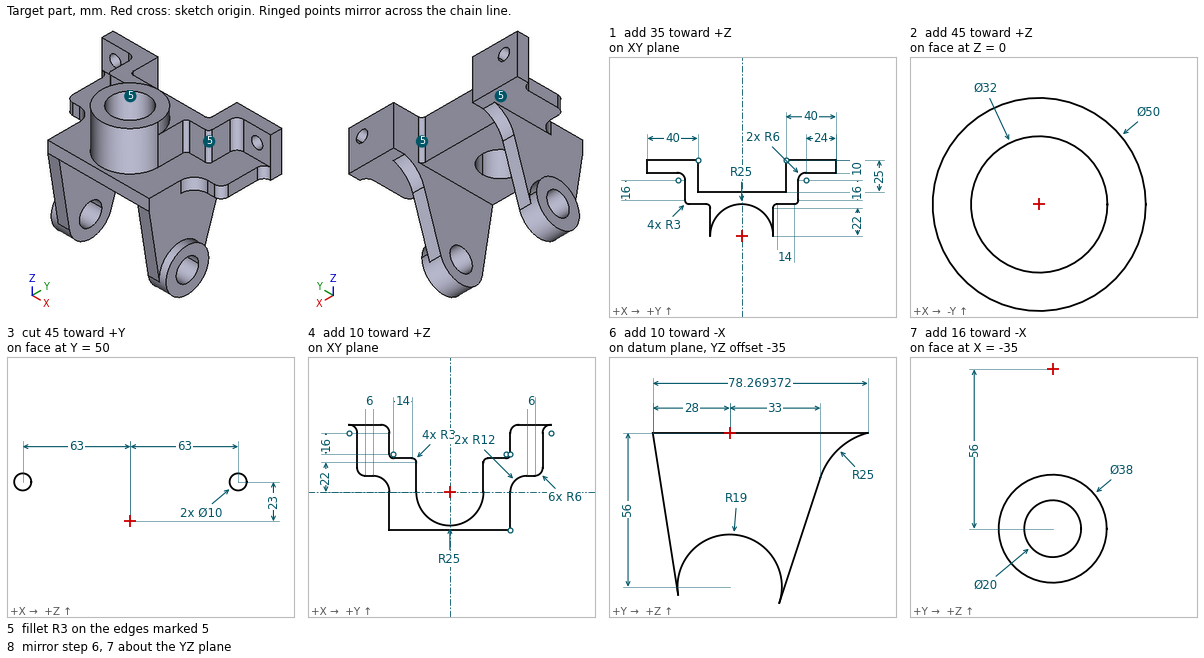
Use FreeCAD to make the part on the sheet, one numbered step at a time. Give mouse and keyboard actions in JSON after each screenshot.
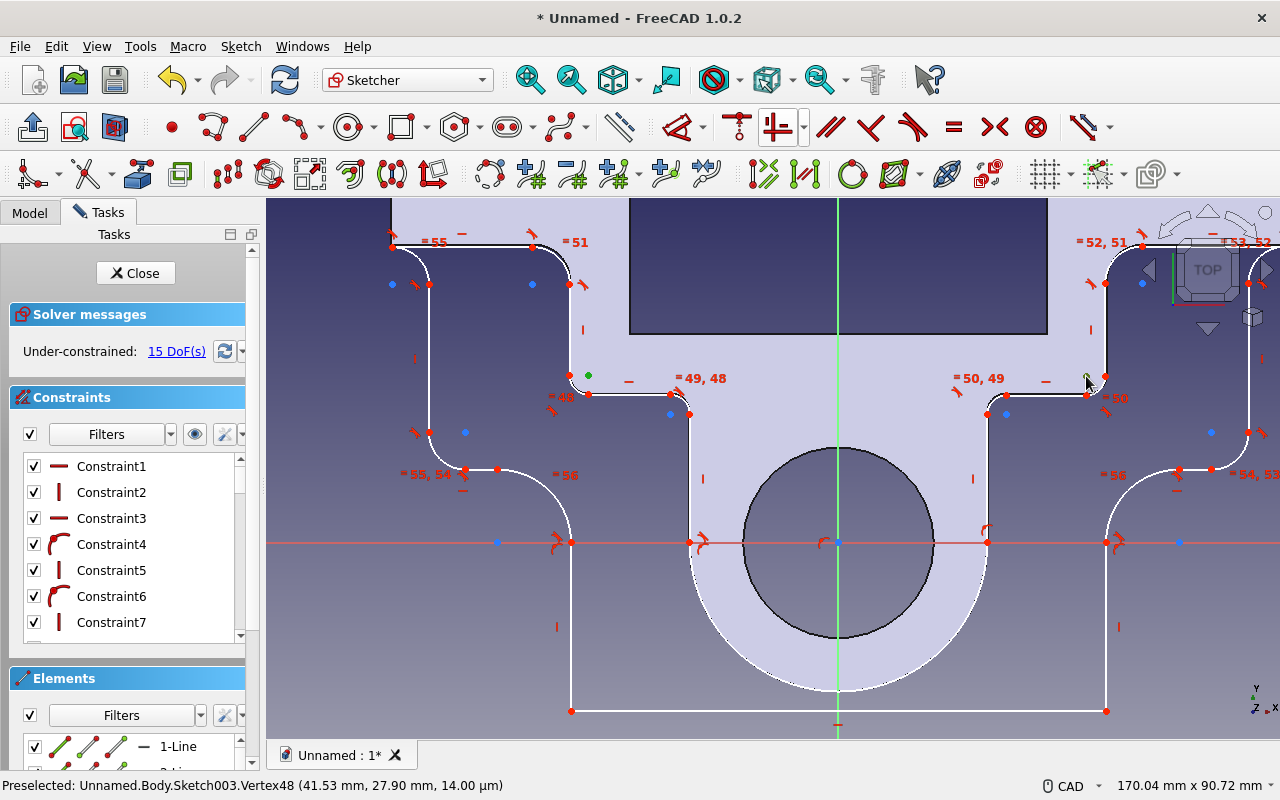
{"action": "left_click", "coordinate": [838, 642]}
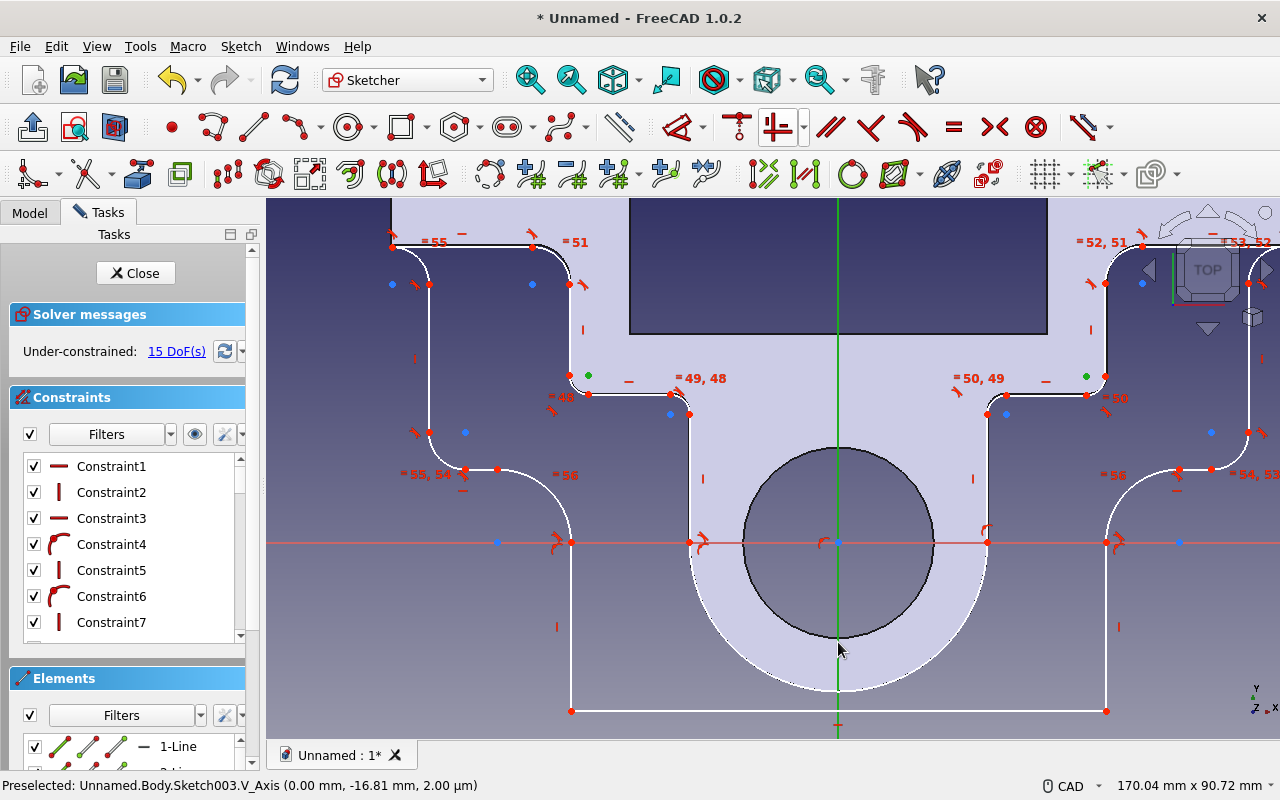
{"action": "left_click", "coordinate": [995, 128]}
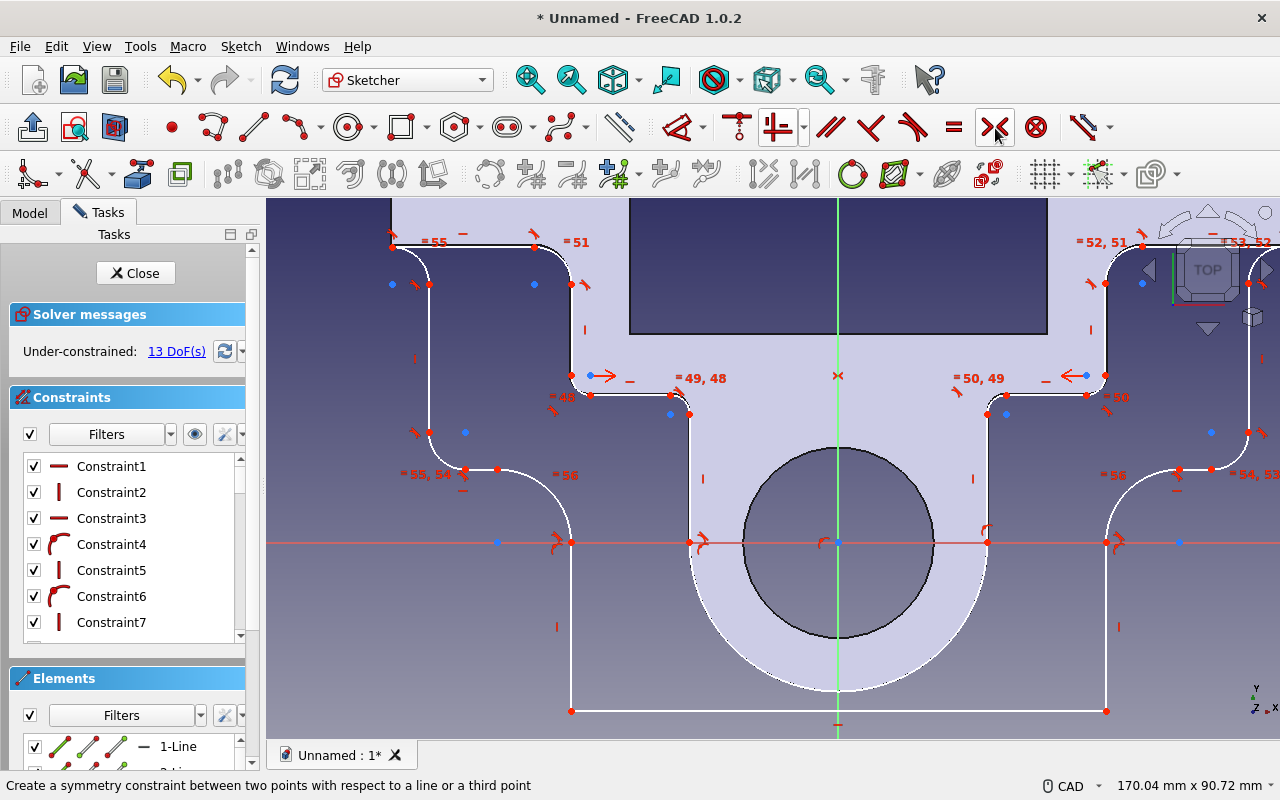
{"action": "scroll", "coordinate": [432, 451], "scroll_direction": "down", "scroll_amount": 2}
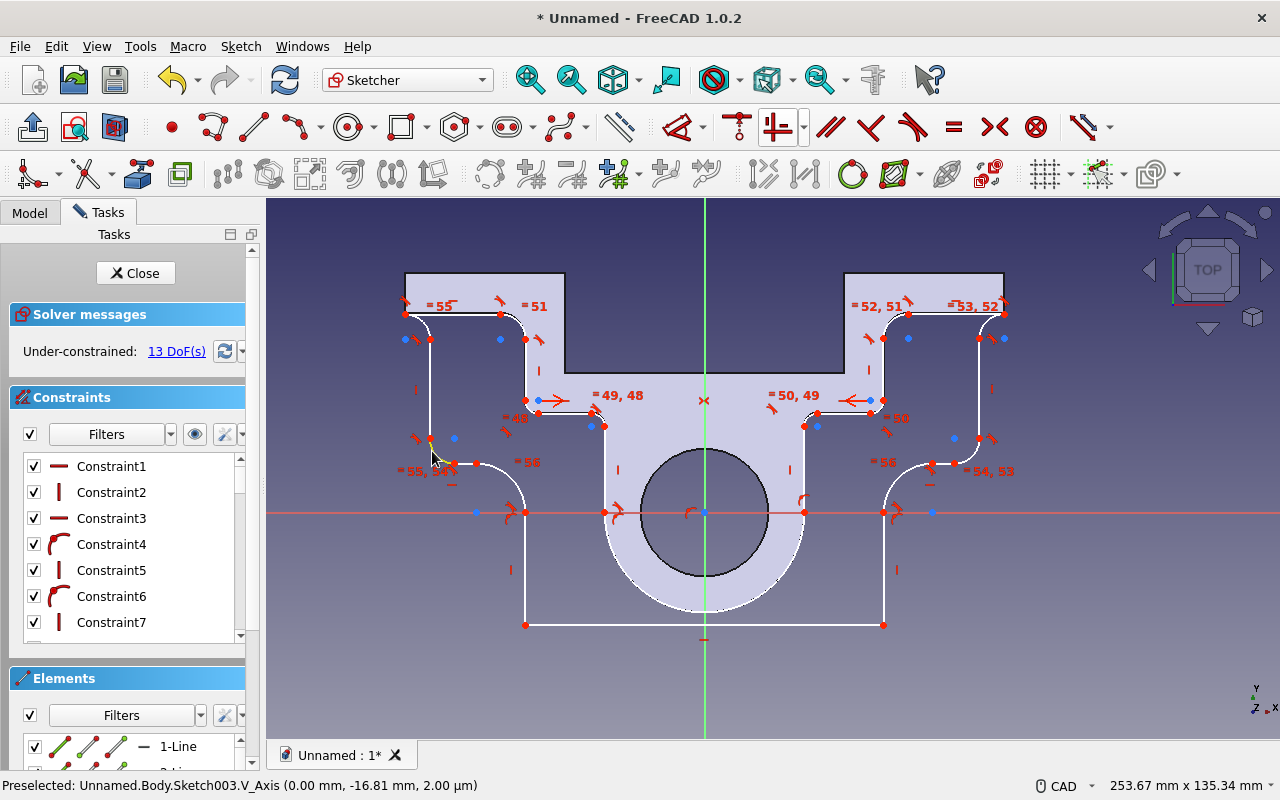
{"action": "left_click", "coordinate": [1004, 339]}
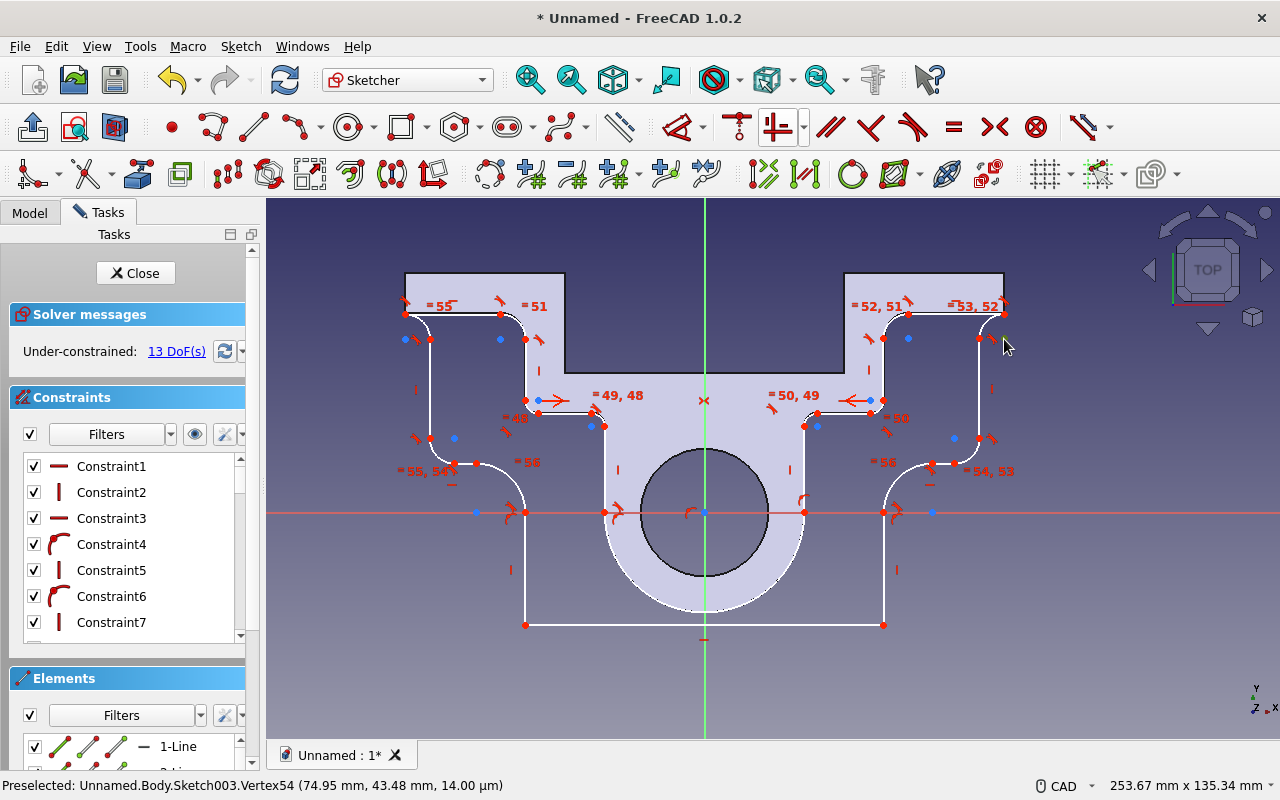
{"action": "left_click", "coordinate": [405, 339]}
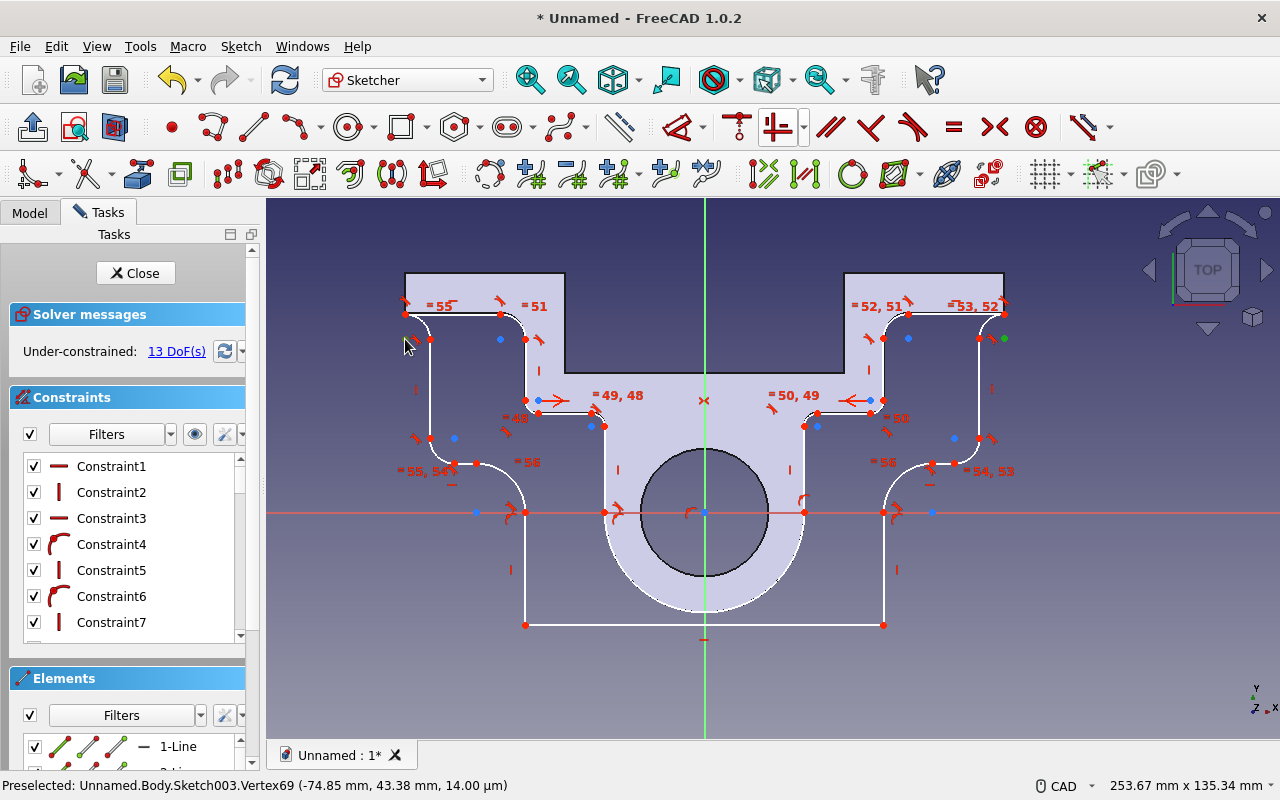
{"action": "left_click", "coordinate": [705, 676]}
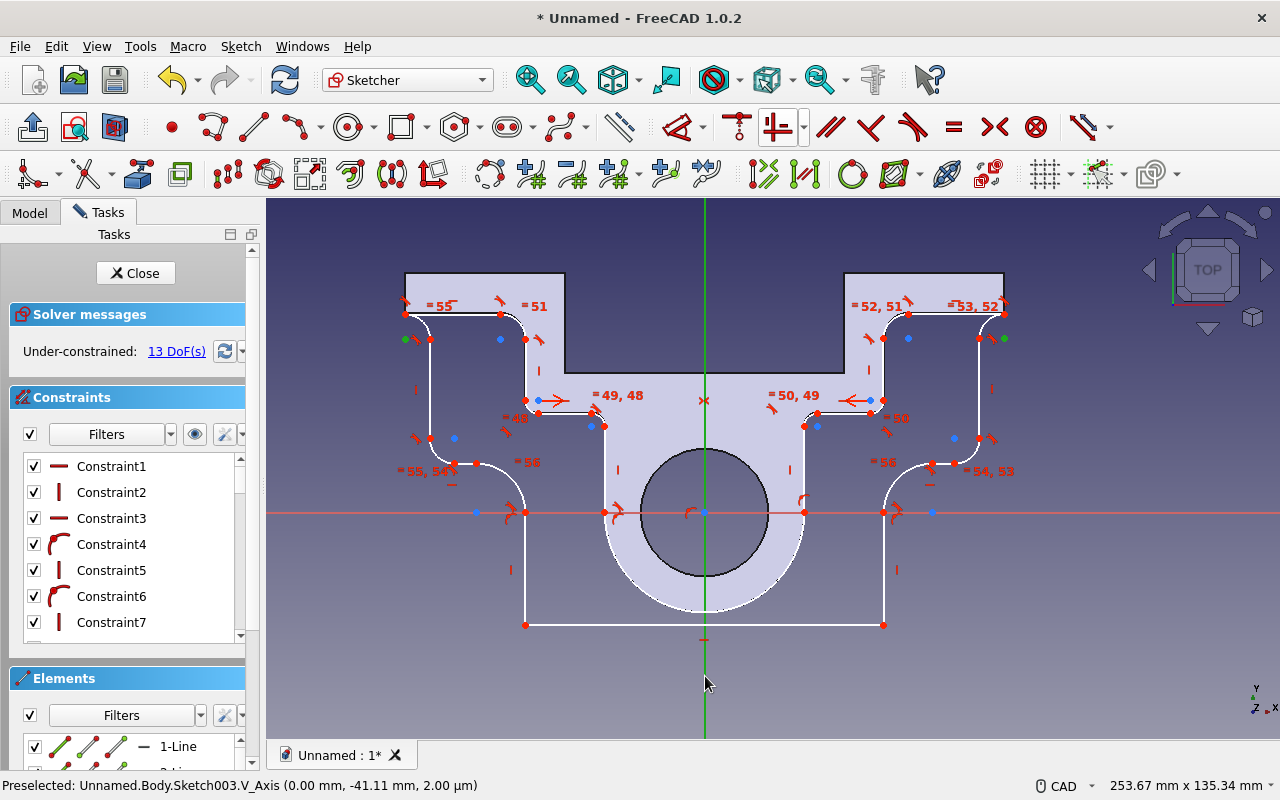
{"action": "left_click", "coordinate": [995, 128]}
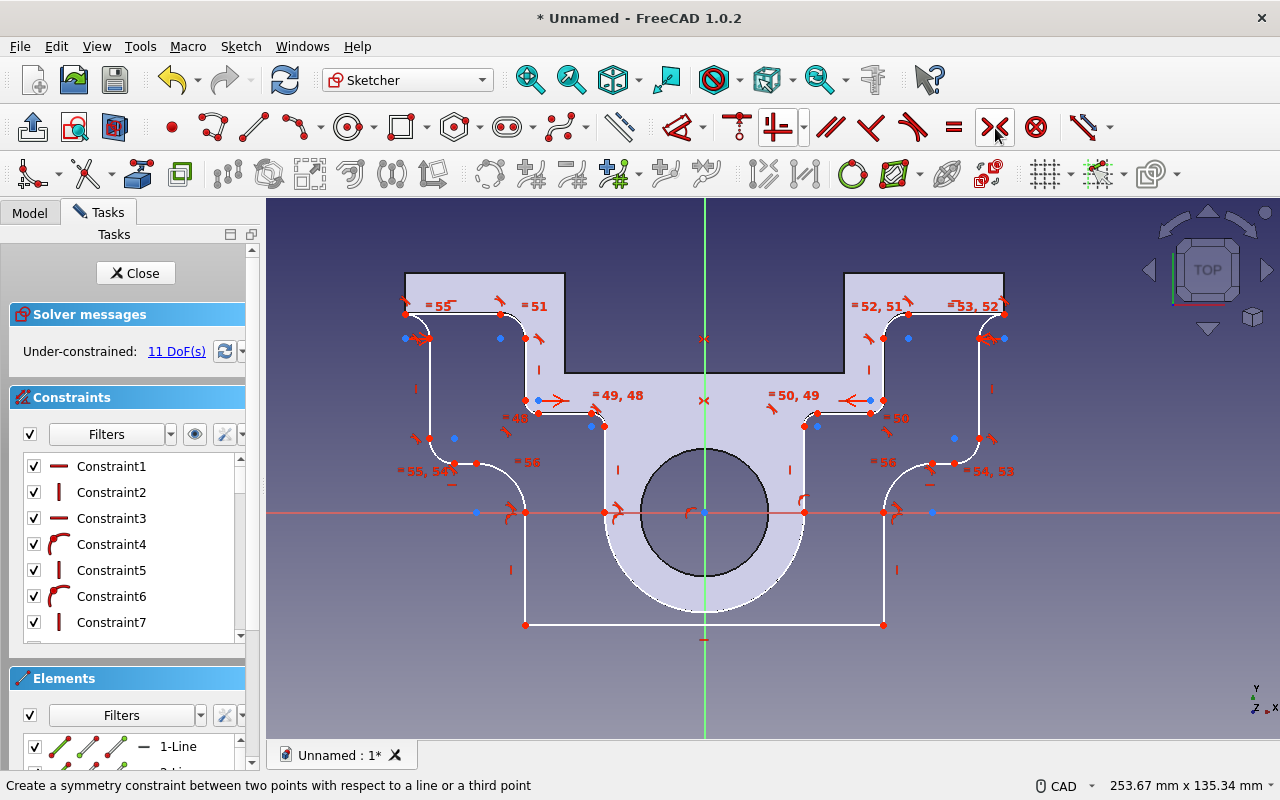
{"action": "left_click", "coordinate": [884, 401]}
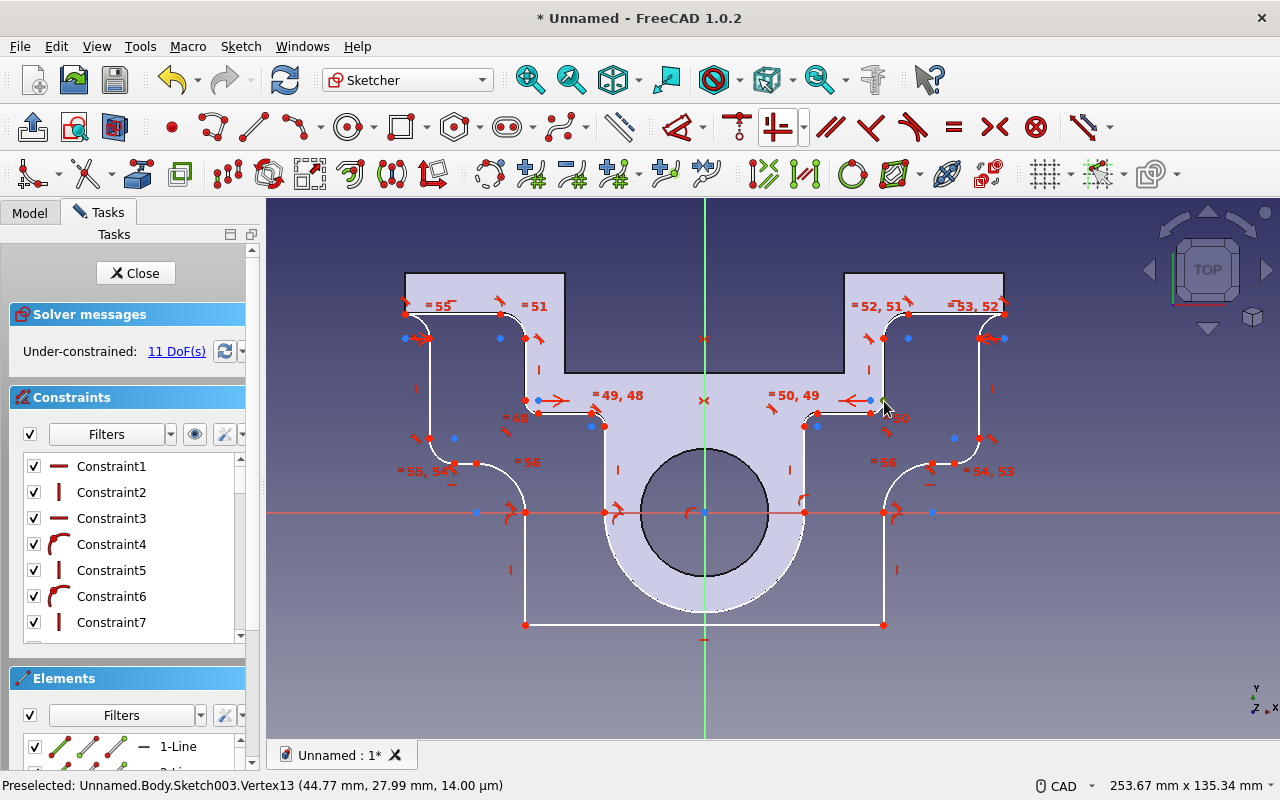
{"action": "left_click", "coordinate": [884, 625]}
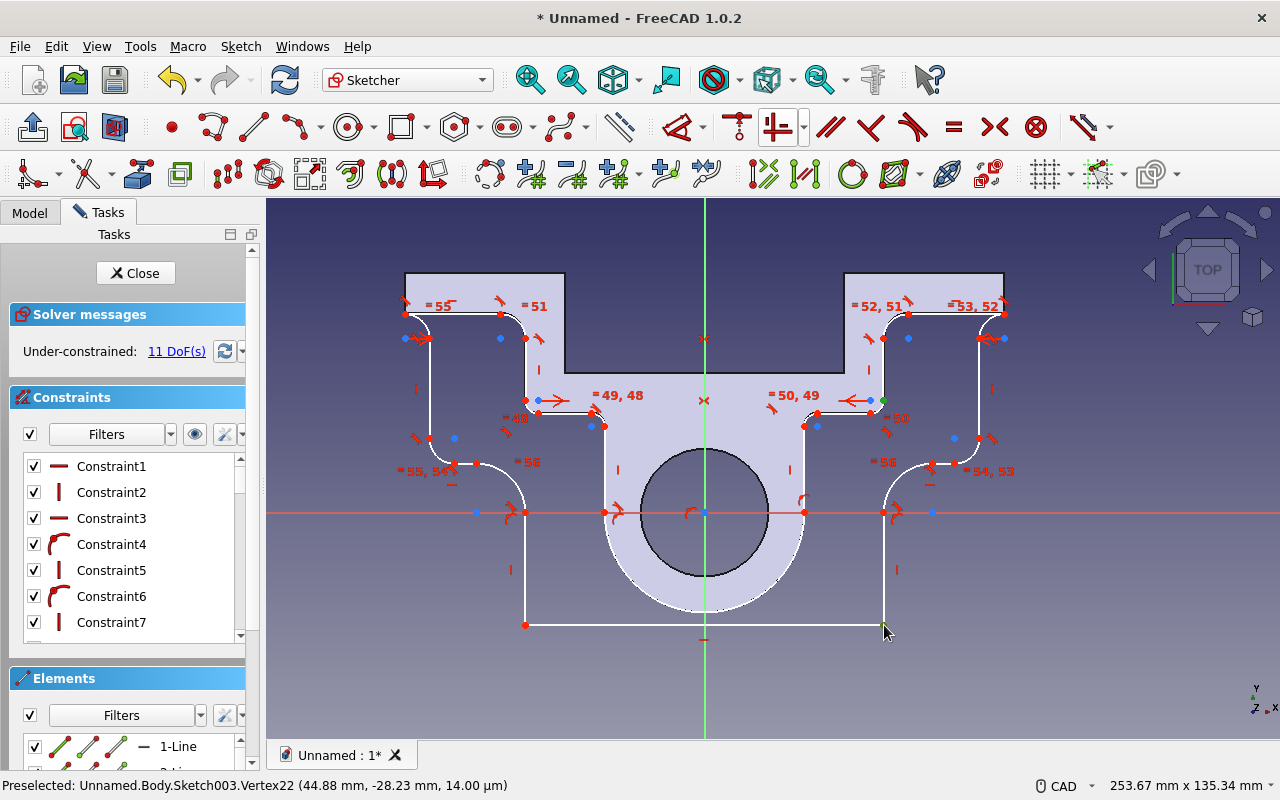
{"action": "left_click", "coordinate": [353, 513]}